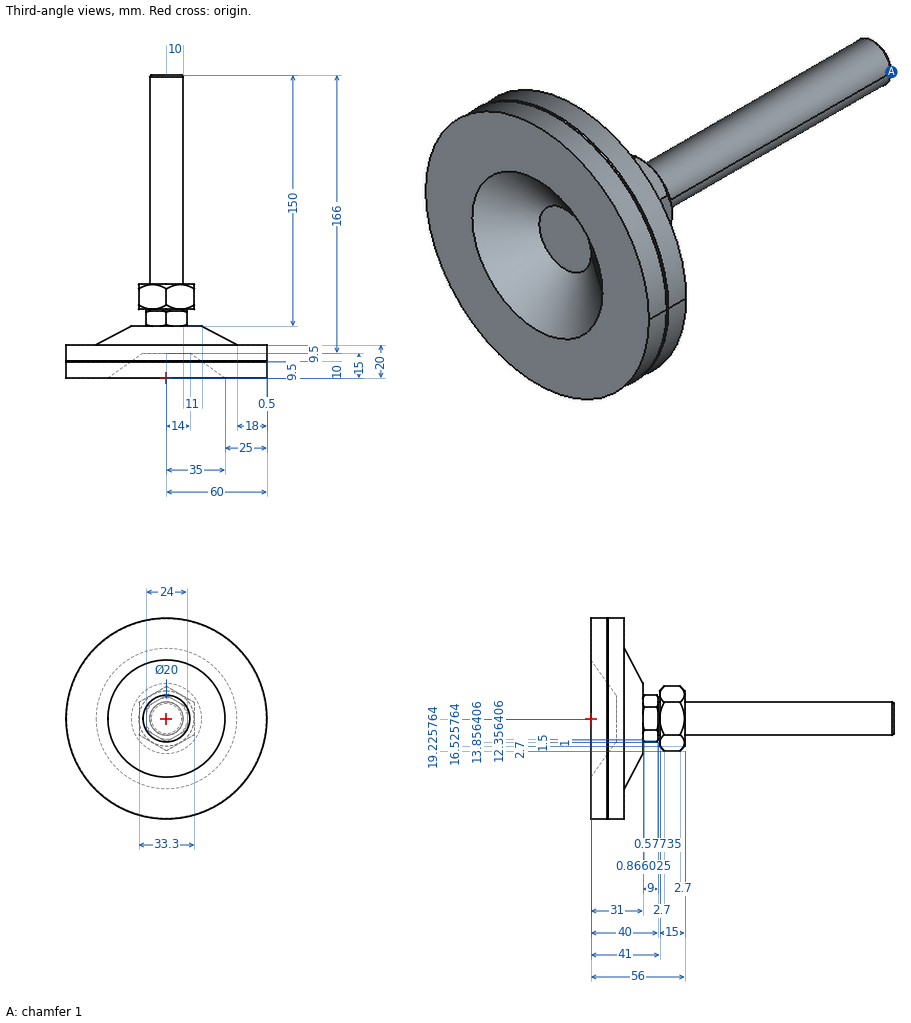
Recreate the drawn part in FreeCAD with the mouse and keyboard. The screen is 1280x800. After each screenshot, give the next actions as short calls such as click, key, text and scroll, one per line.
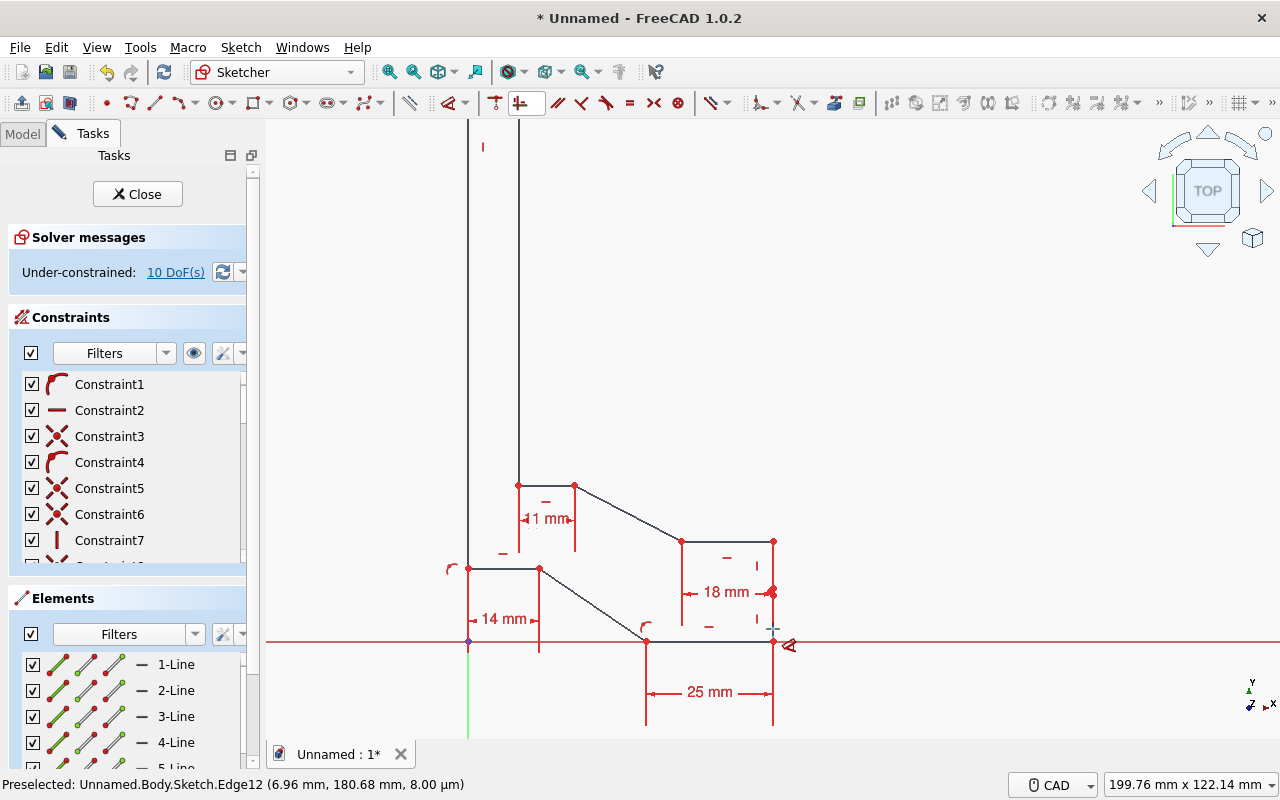
click(773, 628)
click(807, 619)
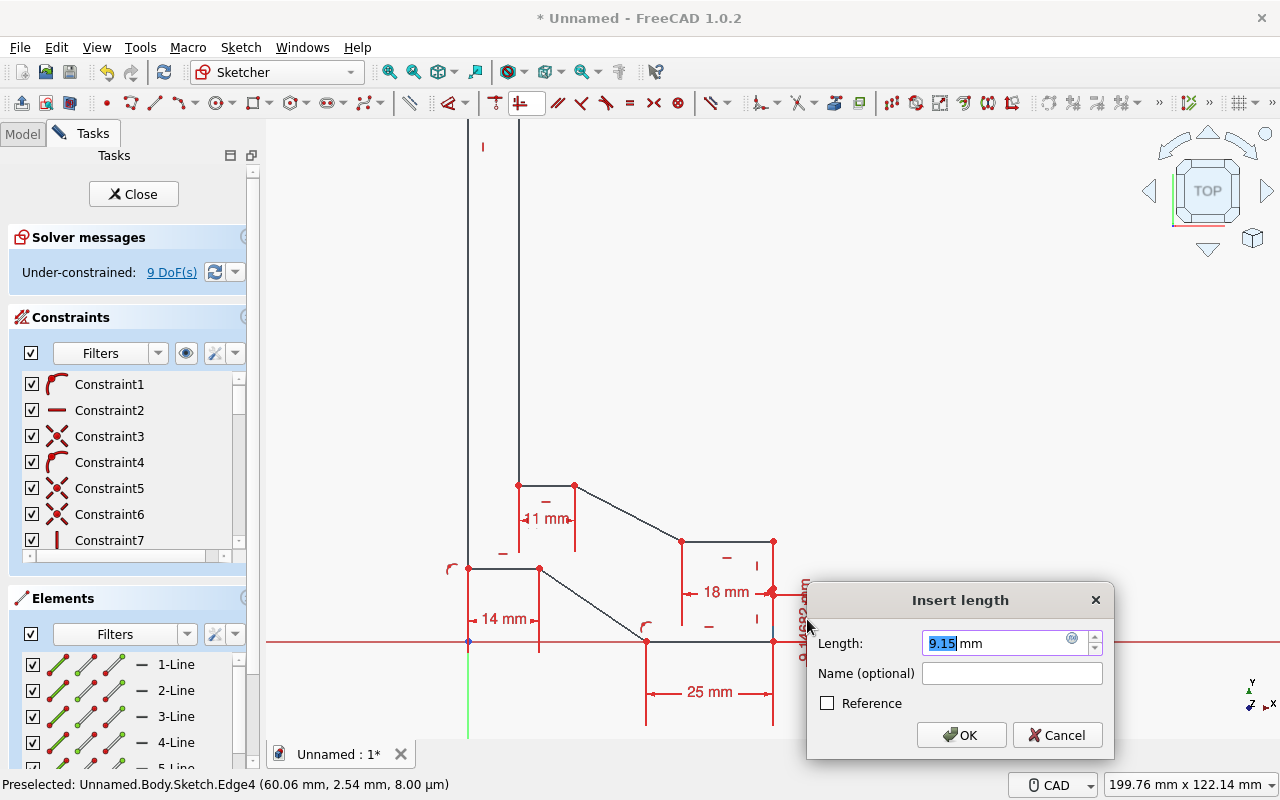
text(9.5)
key(Return)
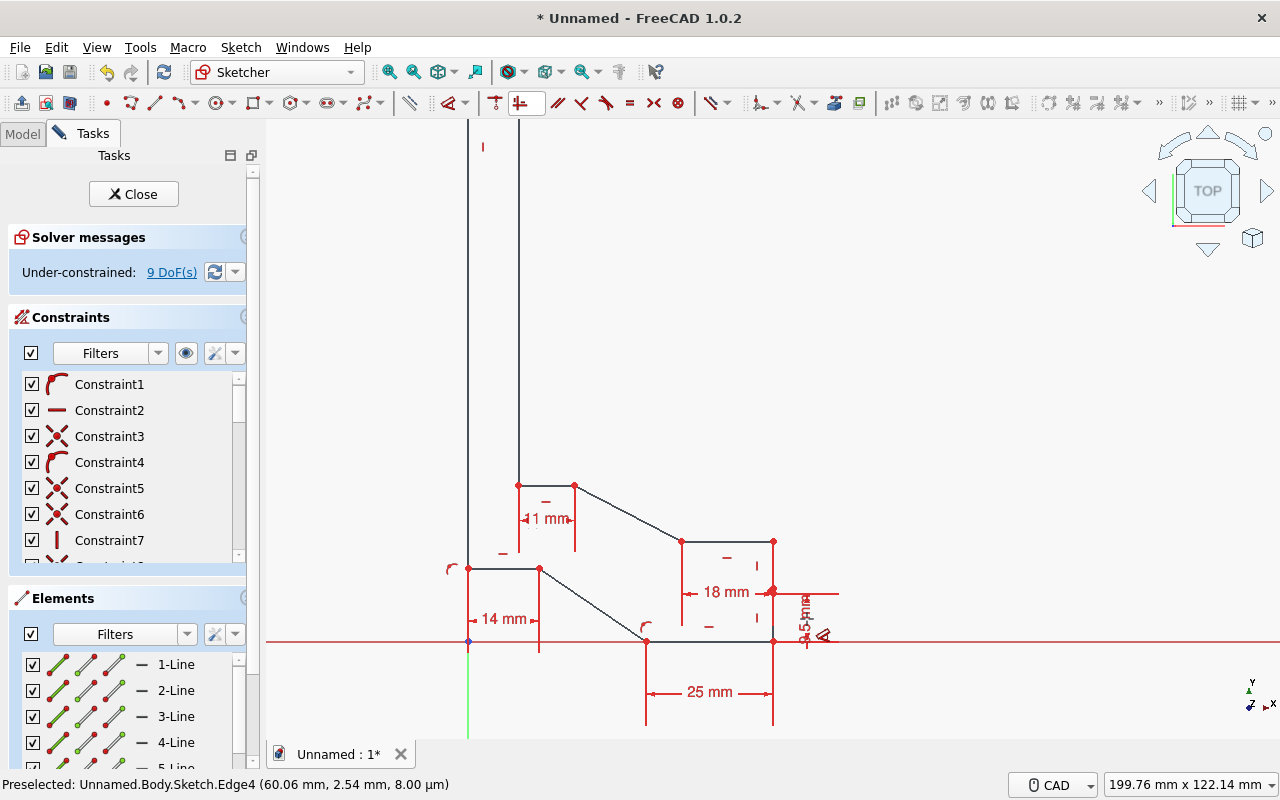
click(773, 575)
click(807, 565)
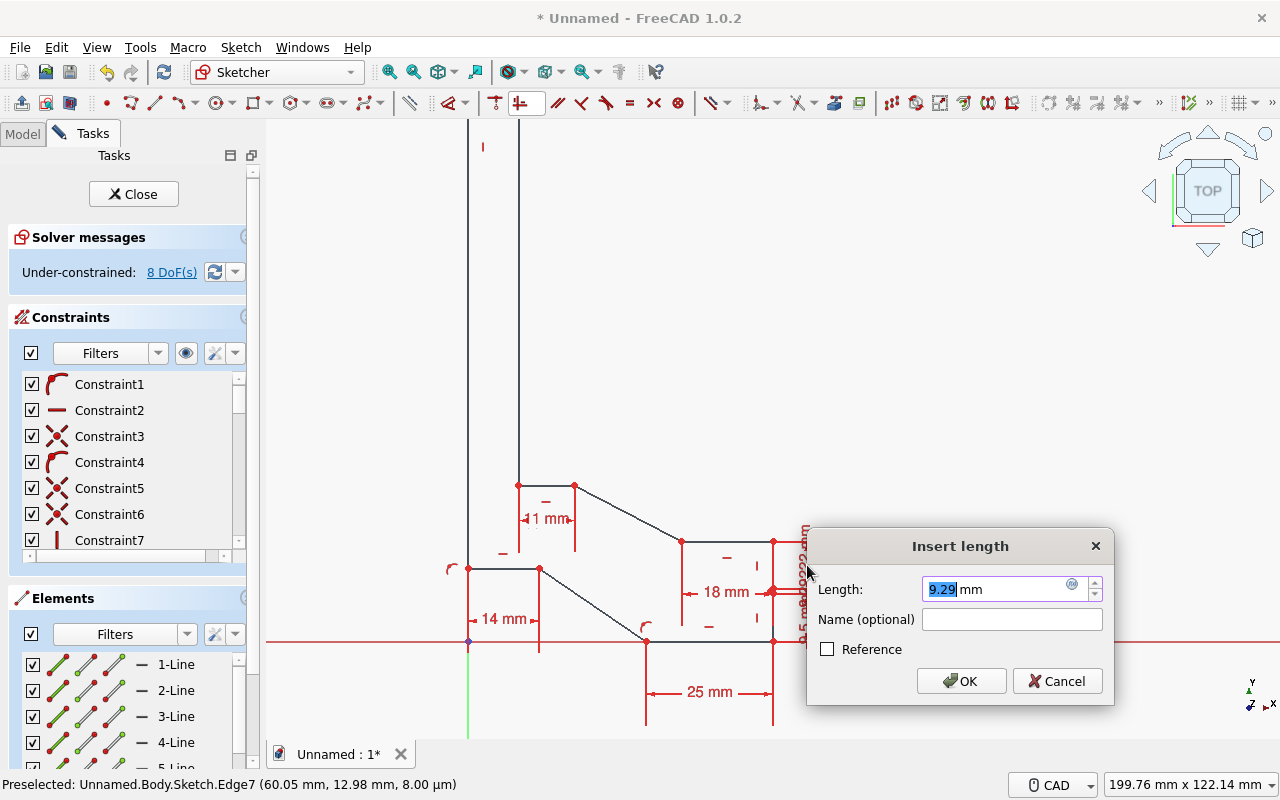
text(9.5)
key(Return)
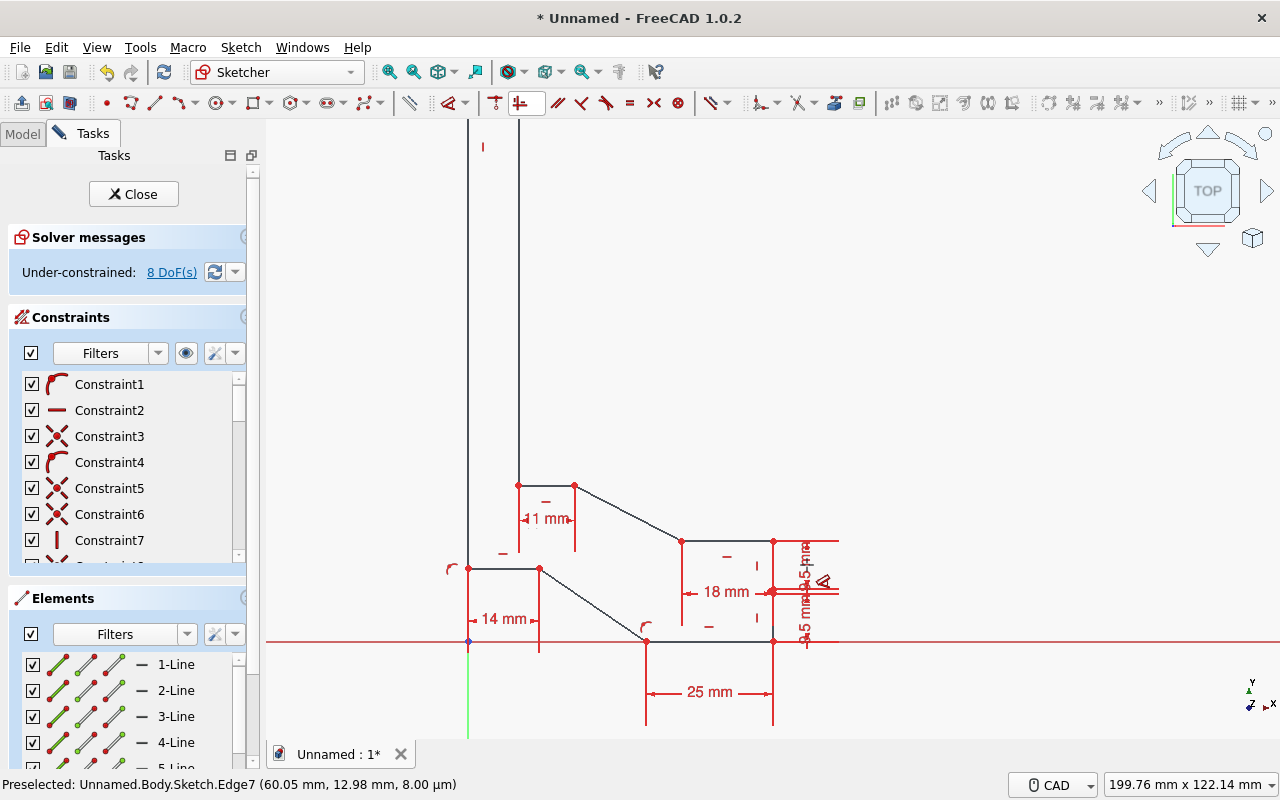
click(519, 258)
click(485, 316)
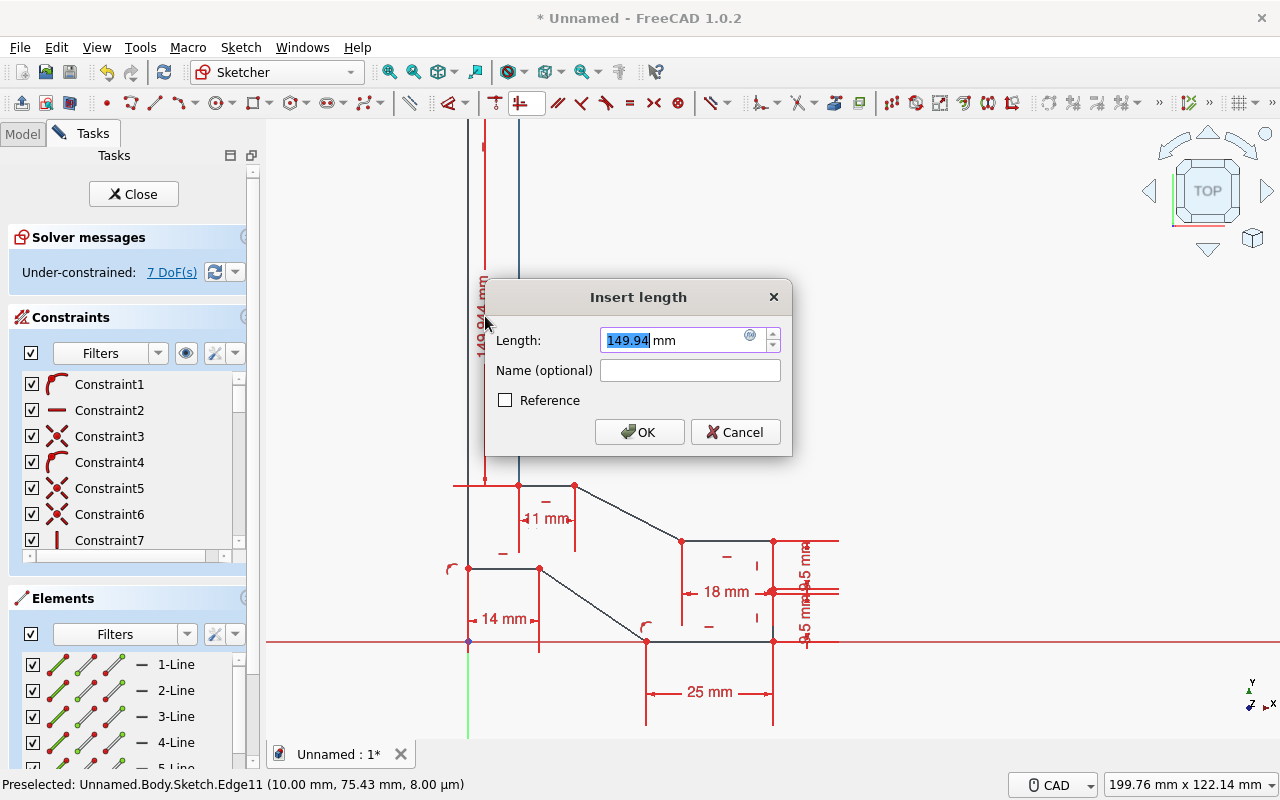
text(150)
key(Return)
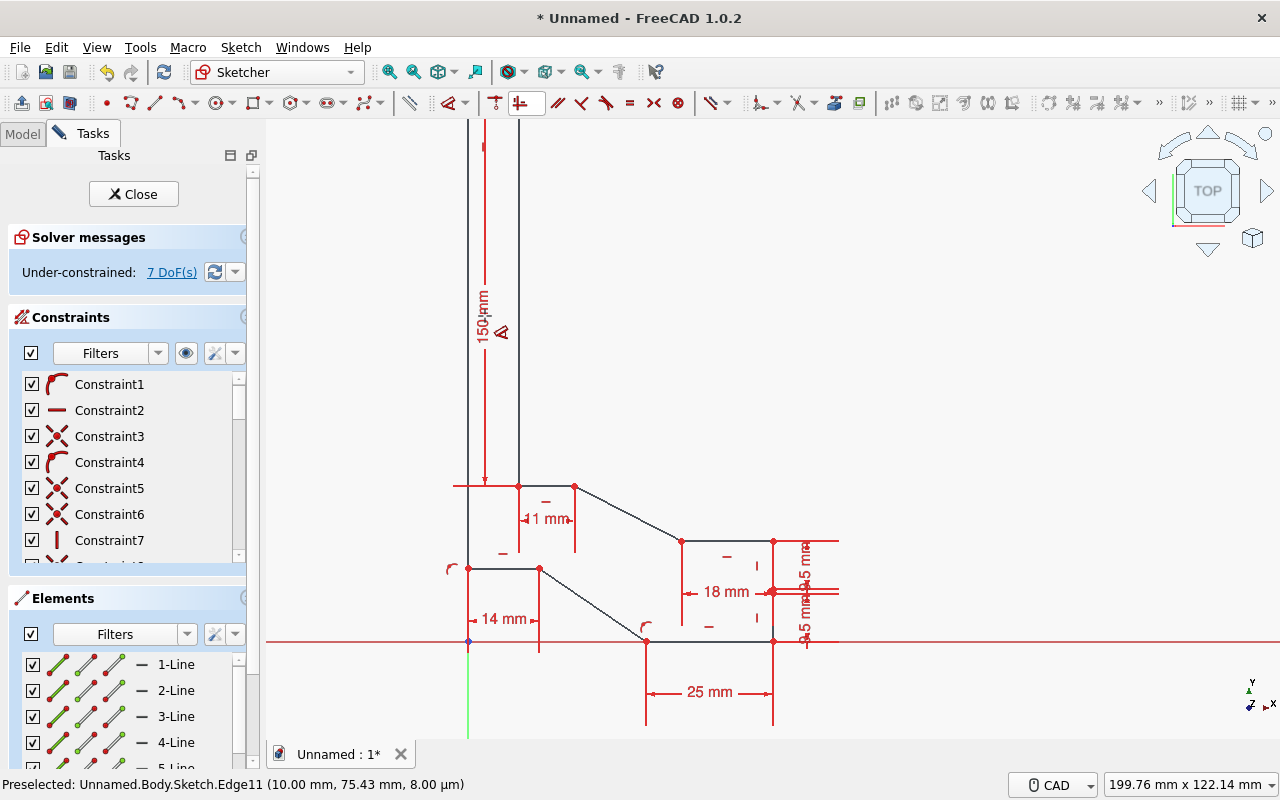
click(468, 316)
click(434, 358)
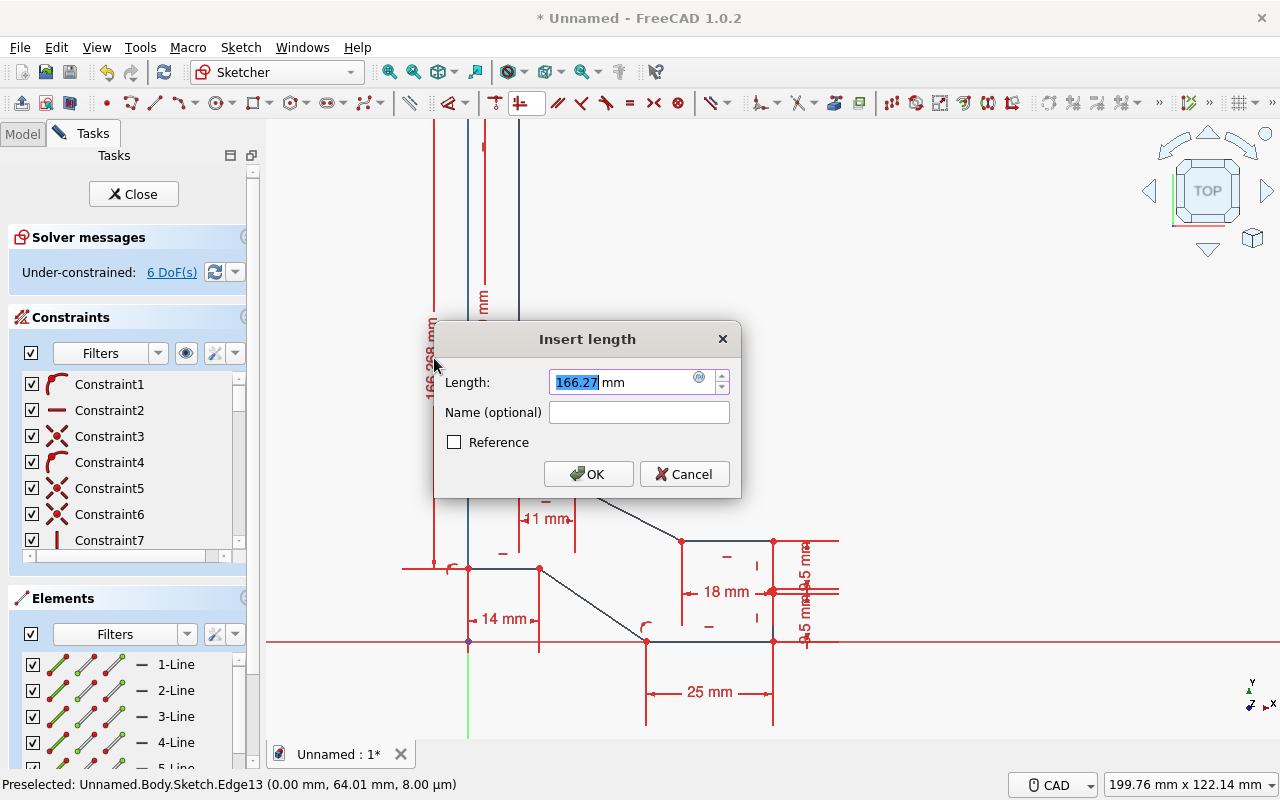
text(166)
key(Return)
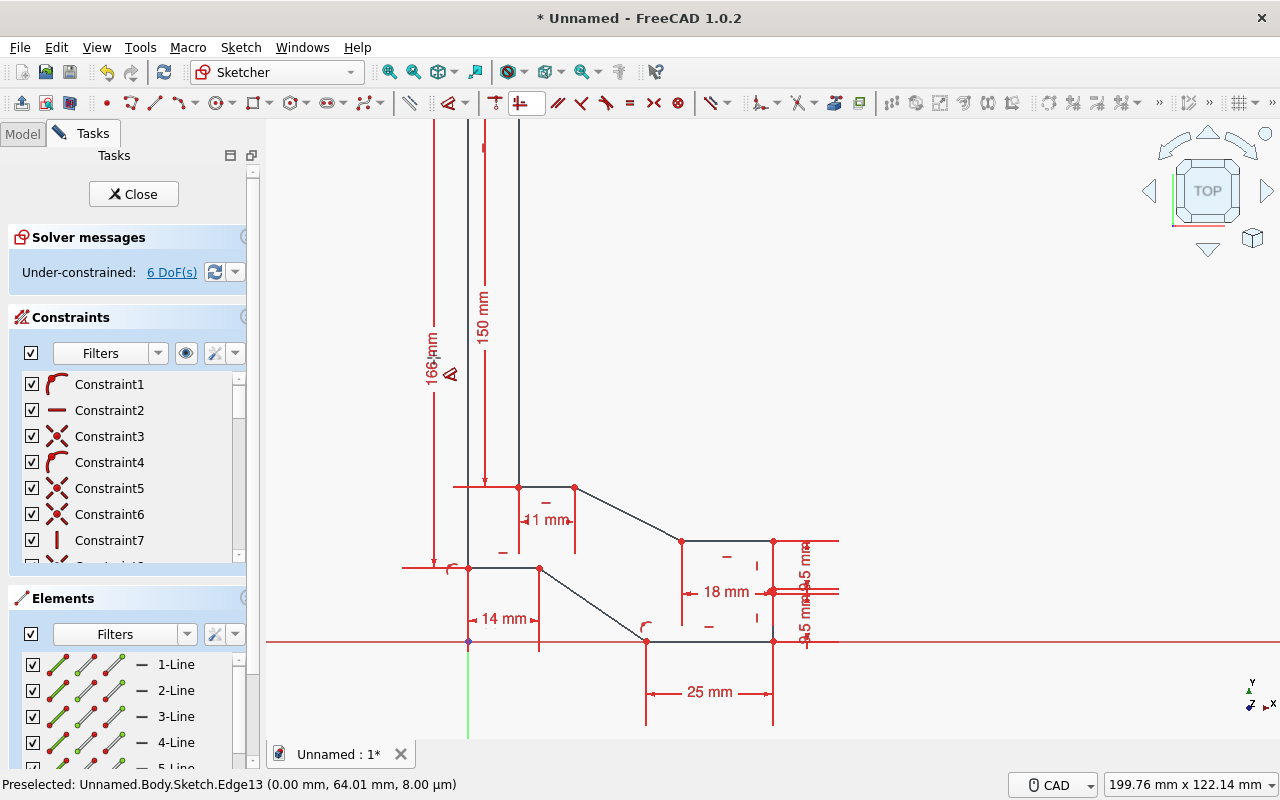
click(468, 568)
click(434, 588)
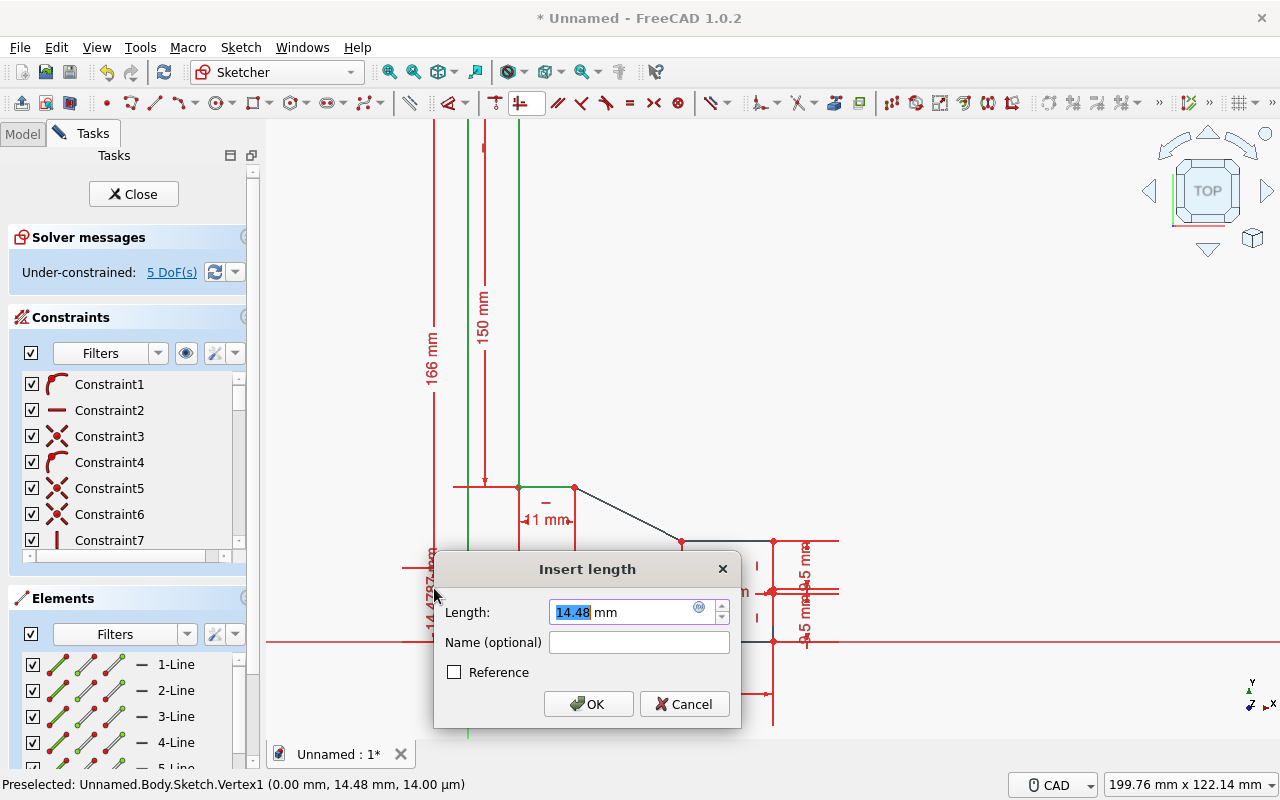
text(15)
key(Return)